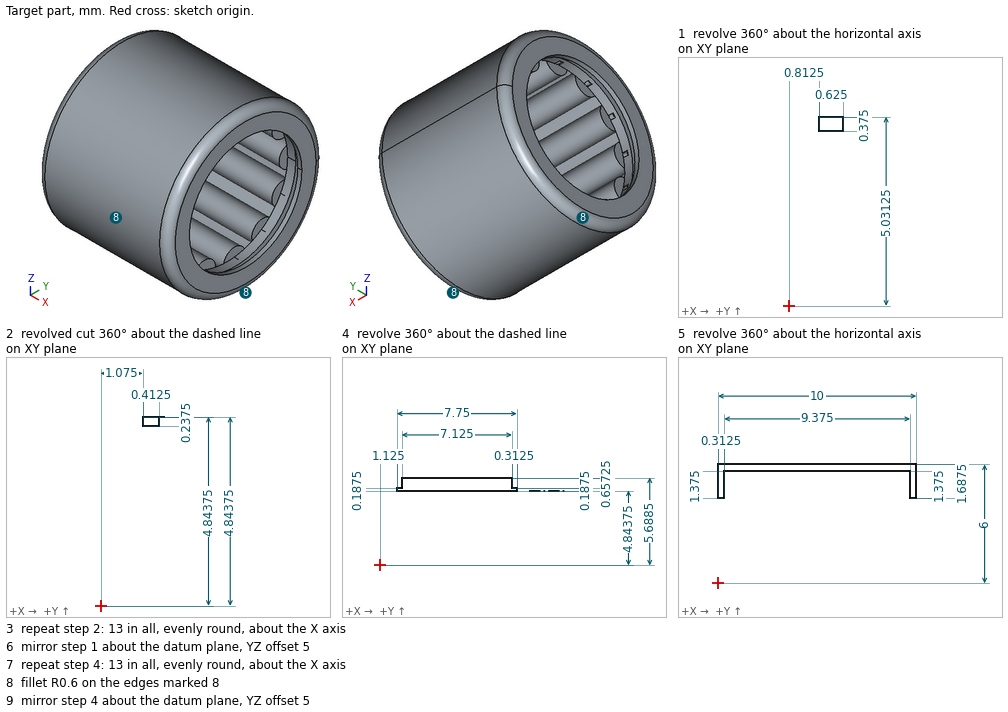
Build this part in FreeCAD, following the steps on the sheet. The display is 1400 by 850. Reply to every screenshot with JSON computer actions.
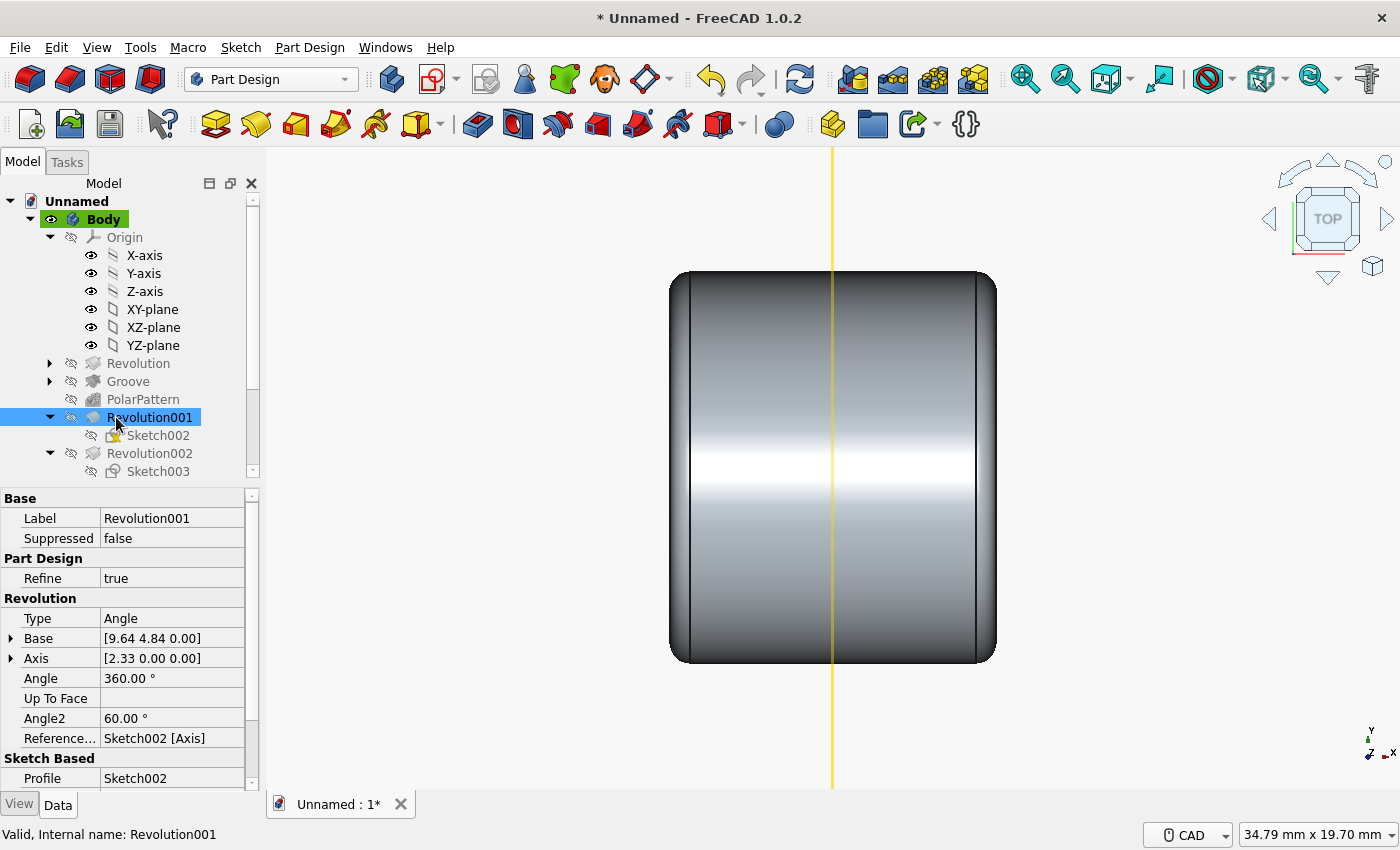
{"action": "left_click", "coordinate": [854, 80]}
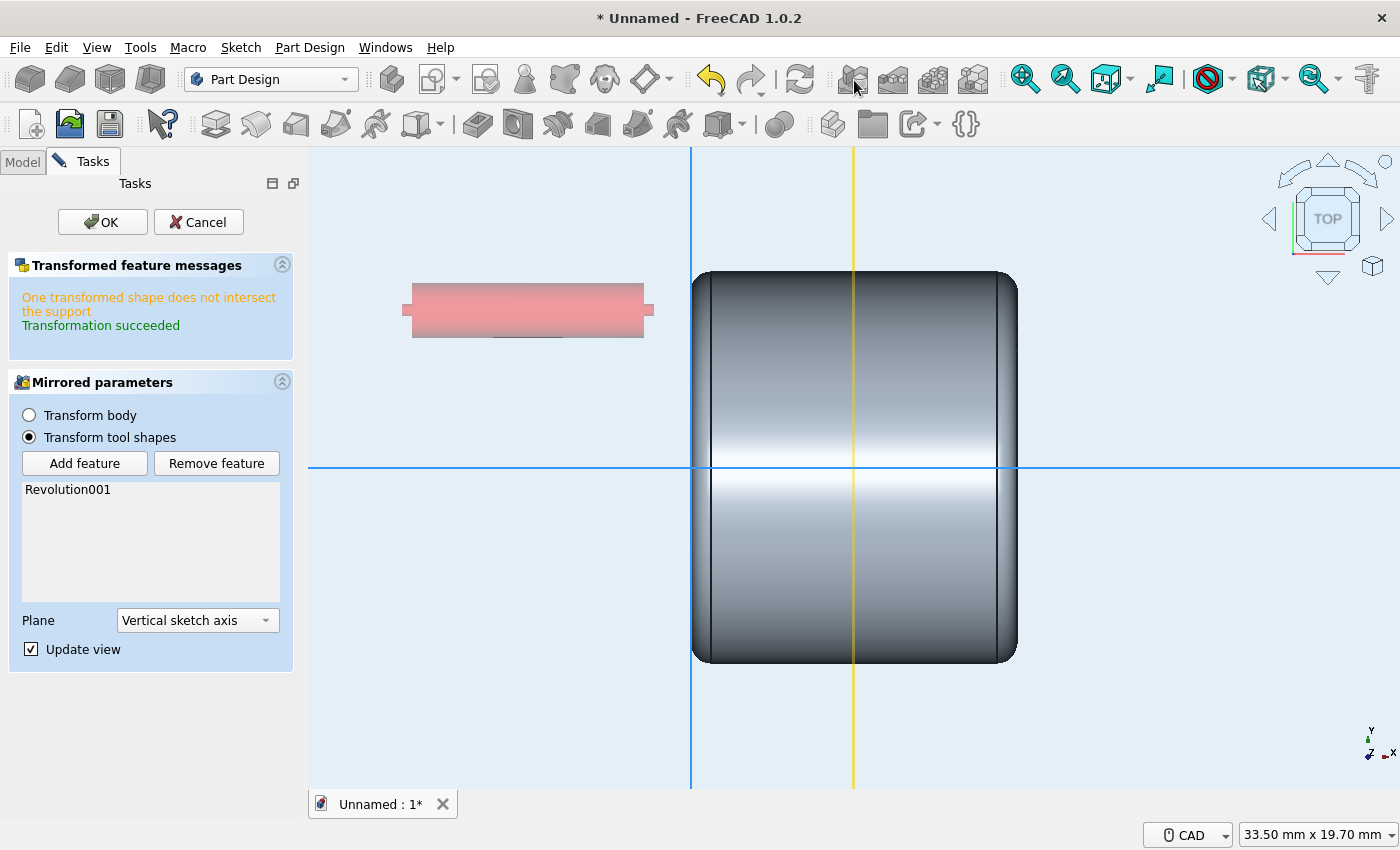
{"action": "left_click", "coordinate": [198, 620]}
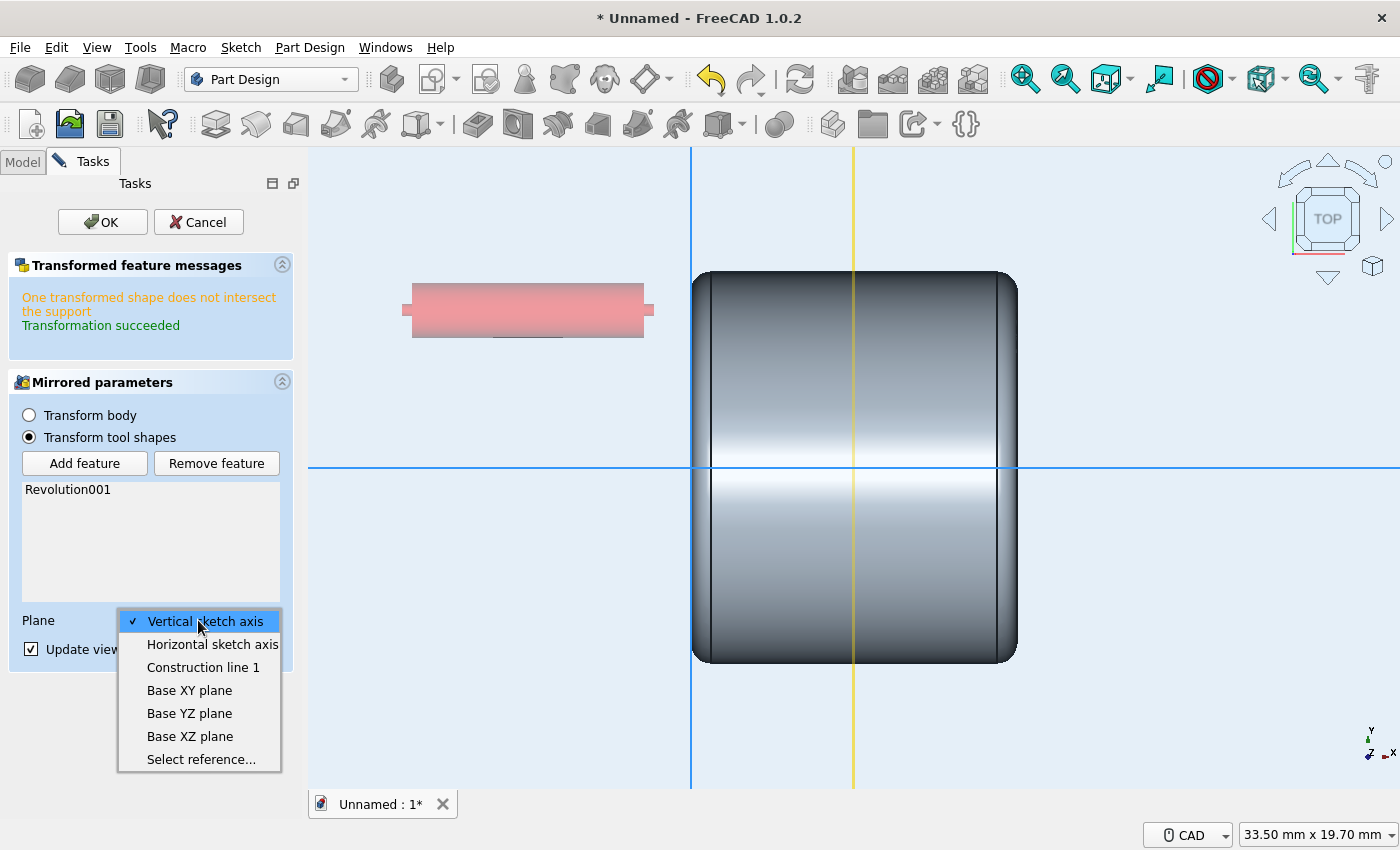
{"action": "left_click", "coordinate": [198, 760]}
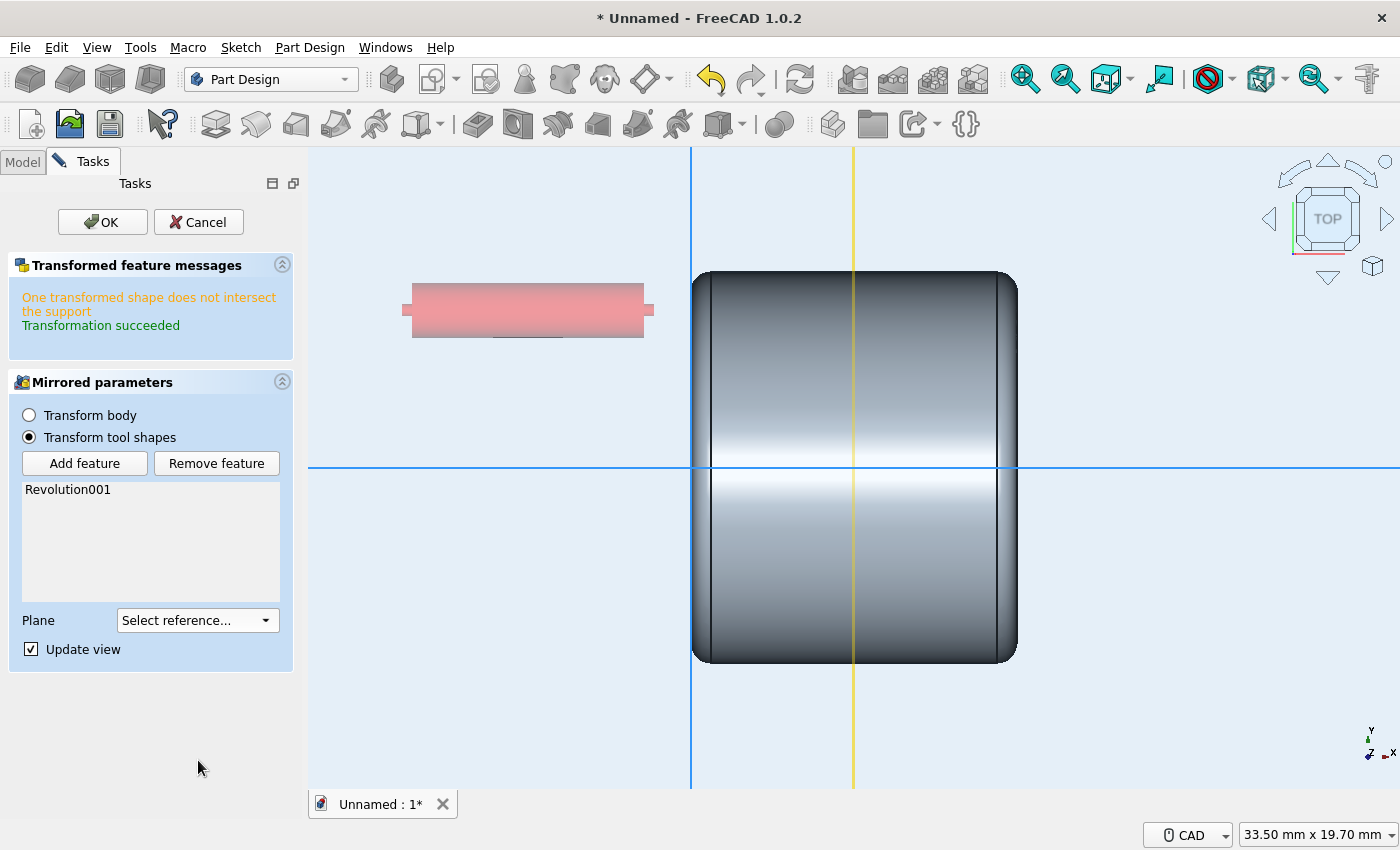
{"action": "left_click", "coordinate": [23, 161]}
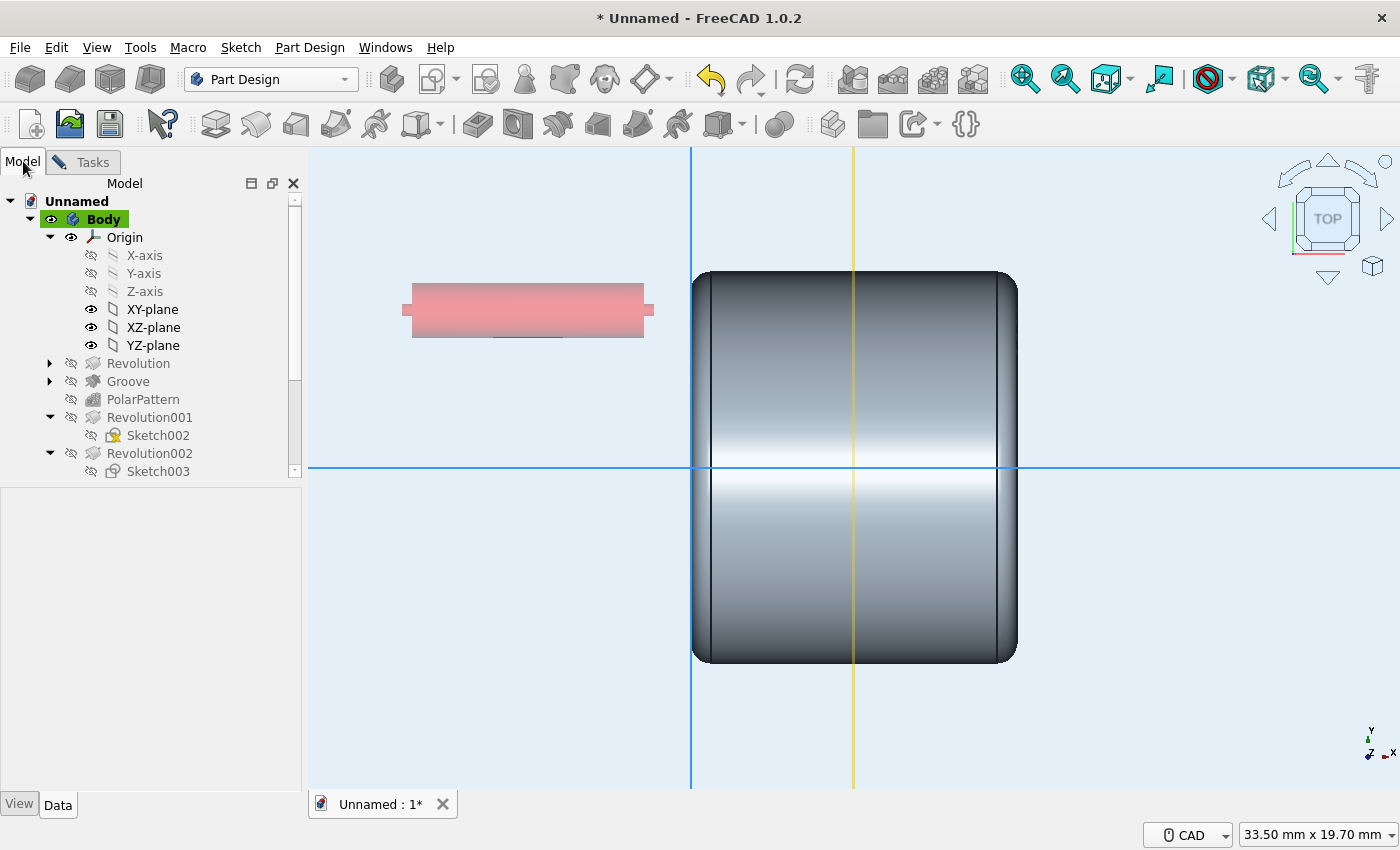
{"action": "scroll", "coordinate": [100, 341], "scroll_direction": "down", "scroll_amount": 3}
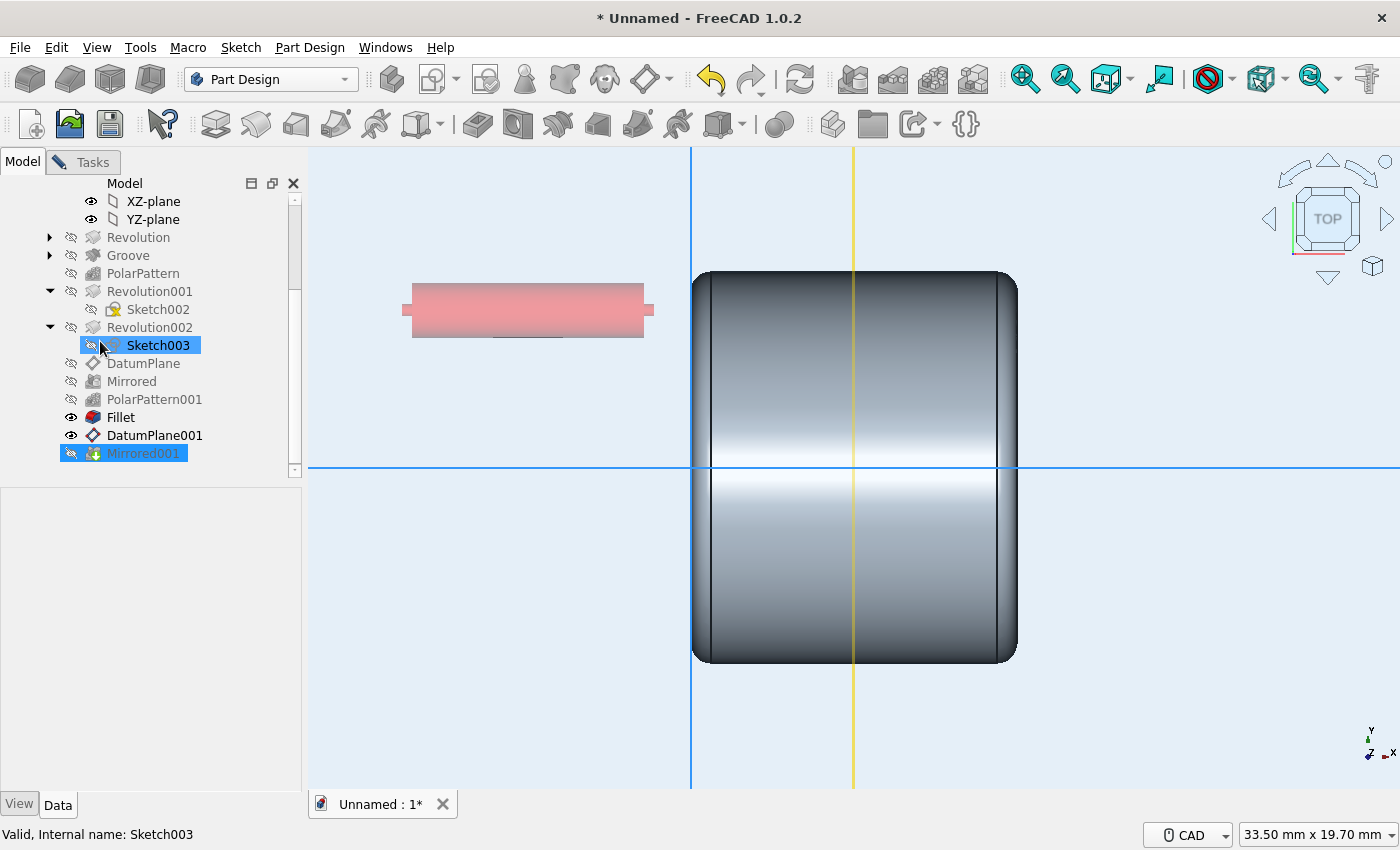
{"action": "left_click", "coordinate": [116, 435]}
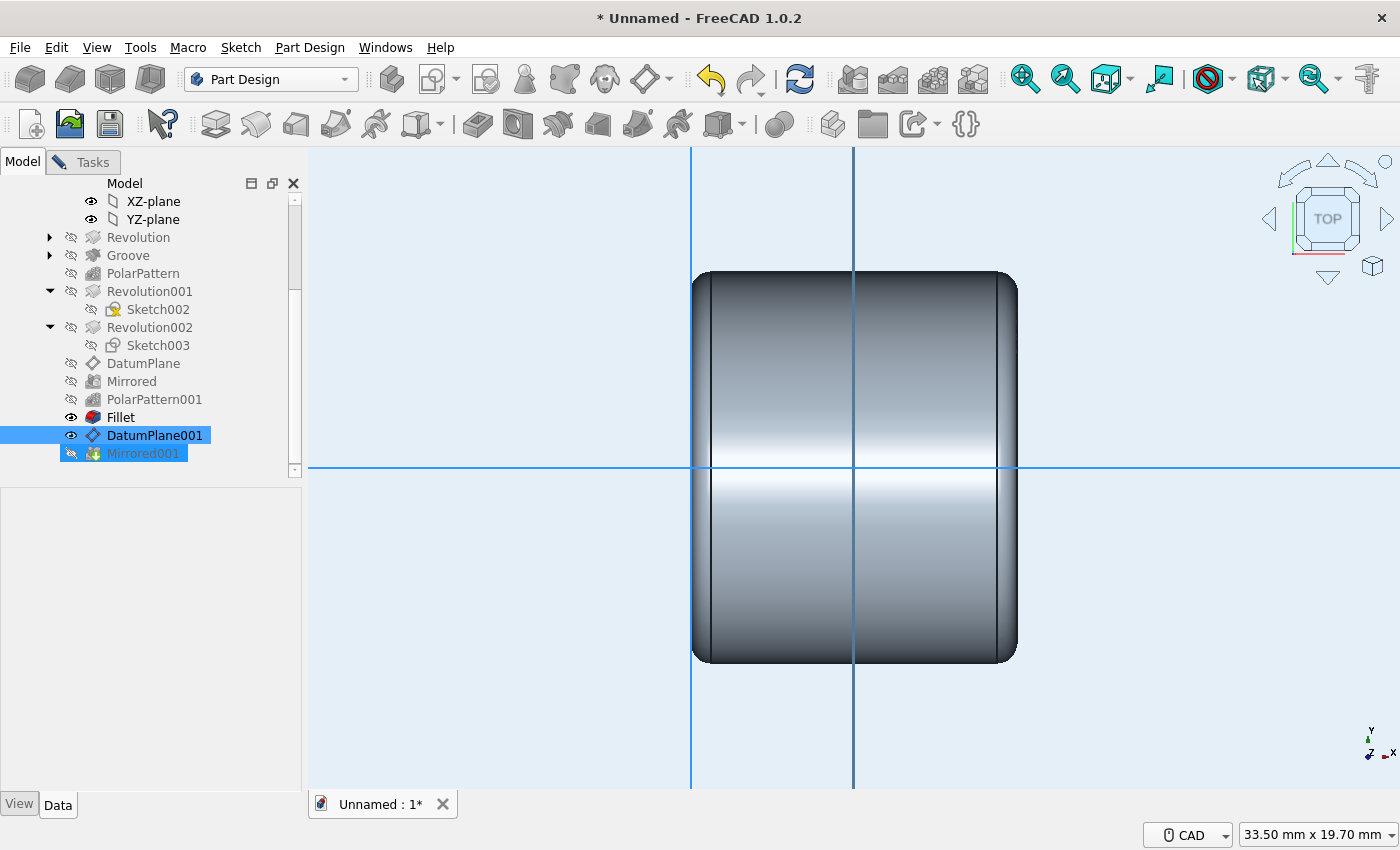
{"action": "left_click", "coordinate": [84, 161]}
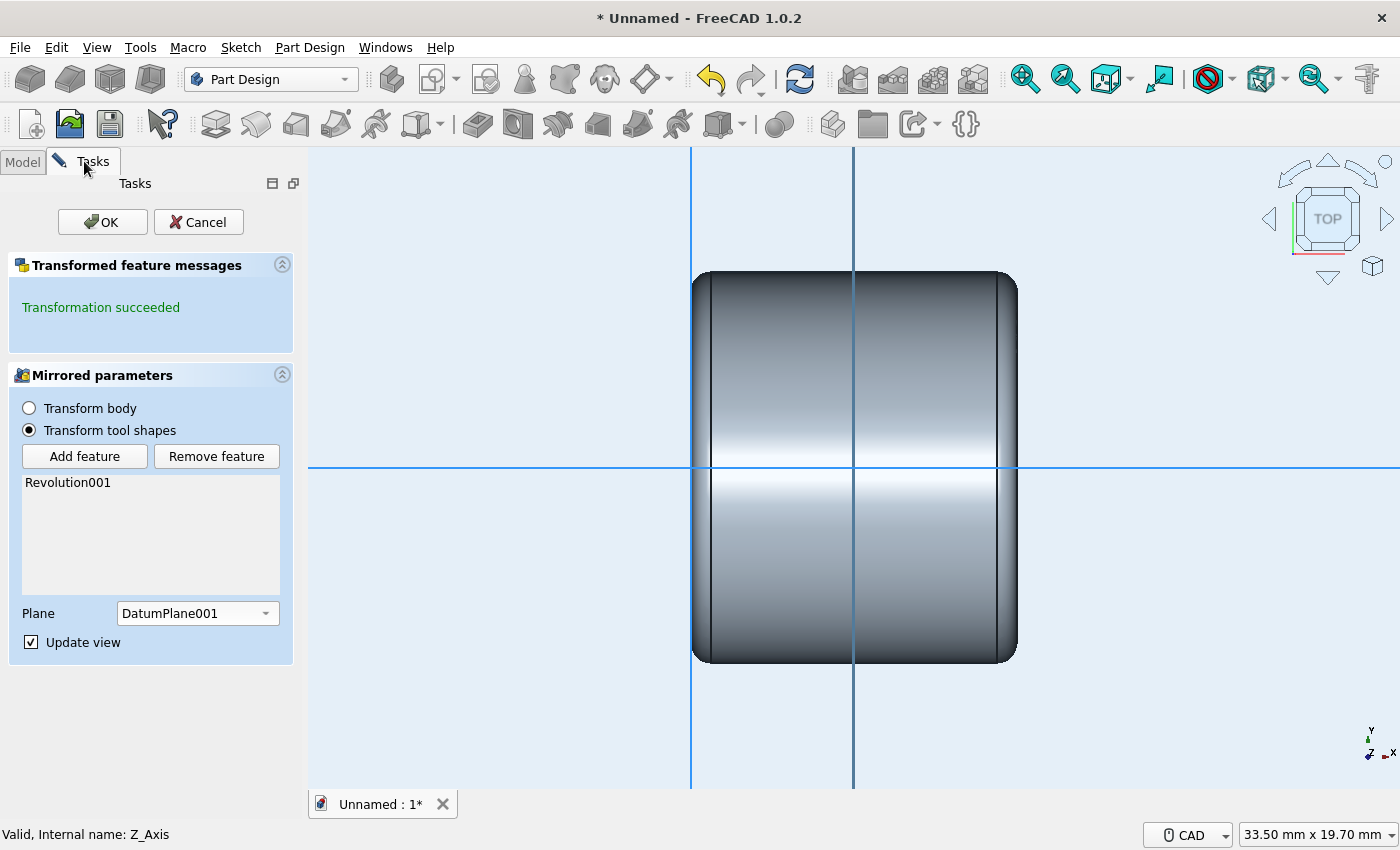
{"action": "left_click", "coordinate": [103, 222]}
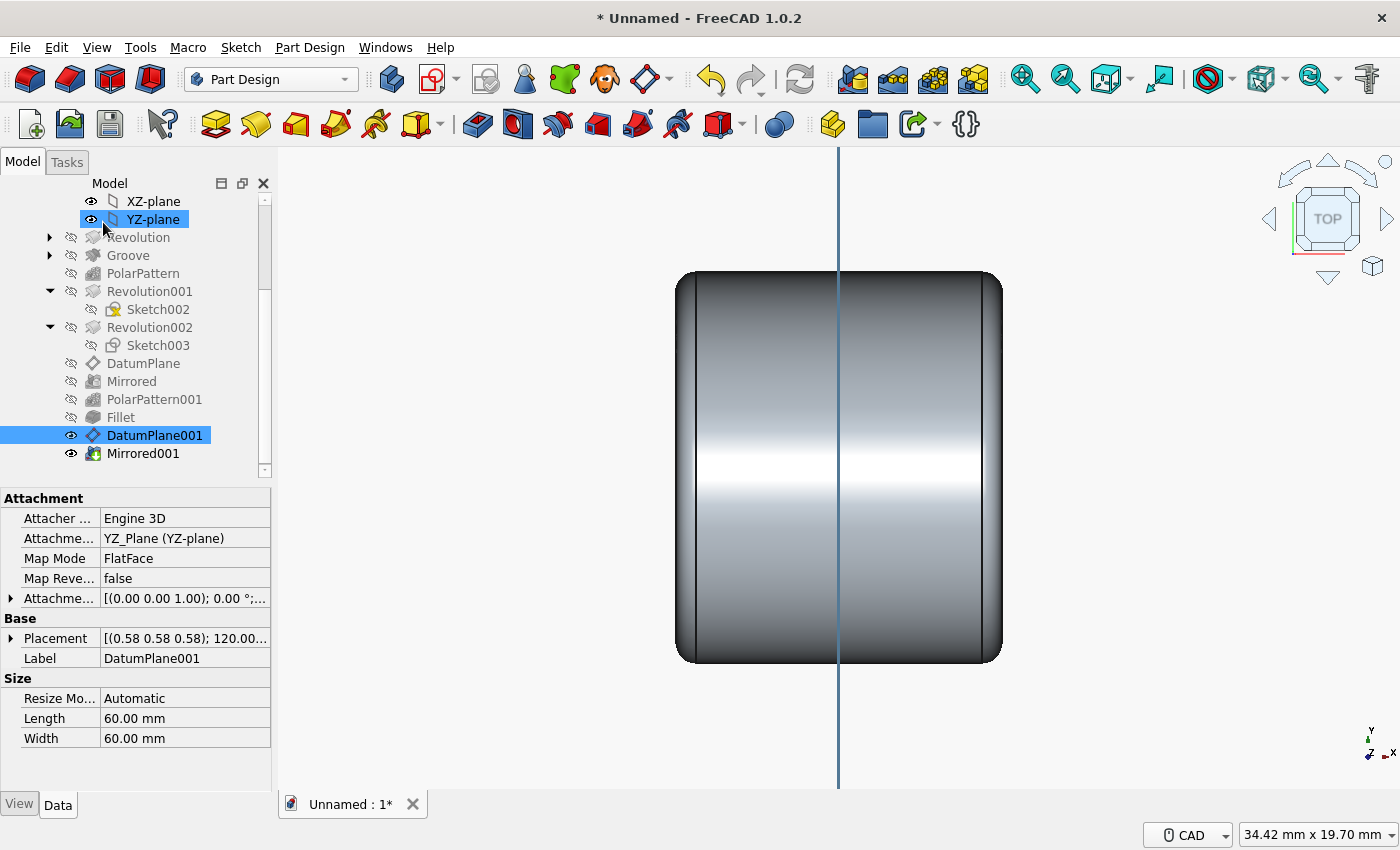
{"action": "left_click", "coordinate": [116, 435]}
{"action": "key", "text": "space"}